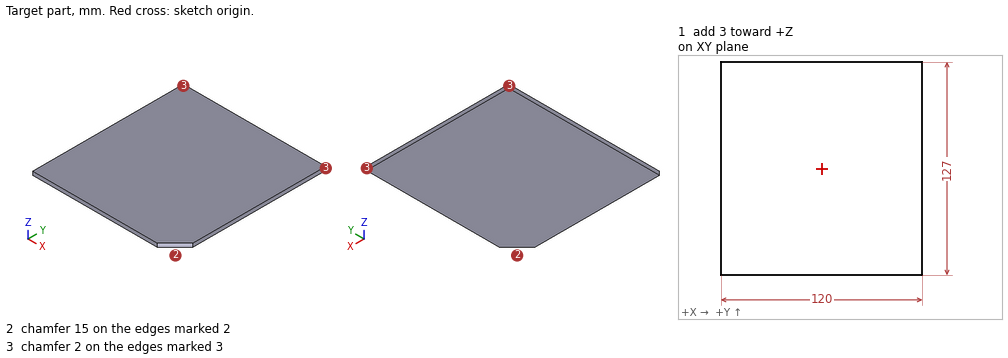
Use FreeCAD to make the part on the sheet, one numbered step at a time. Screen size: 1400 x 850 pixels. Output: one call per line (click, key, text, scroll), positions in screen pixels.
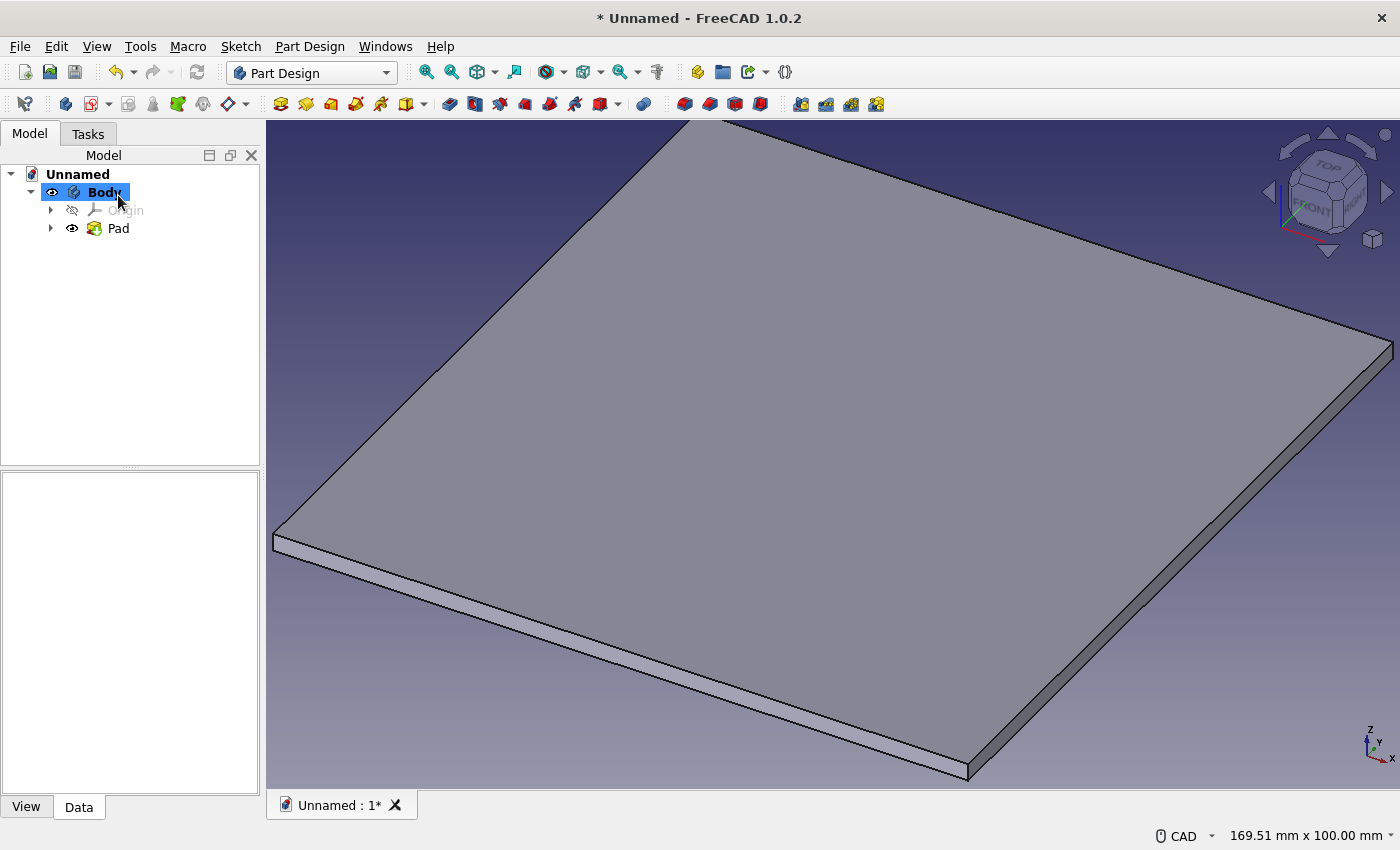
click(427, 72)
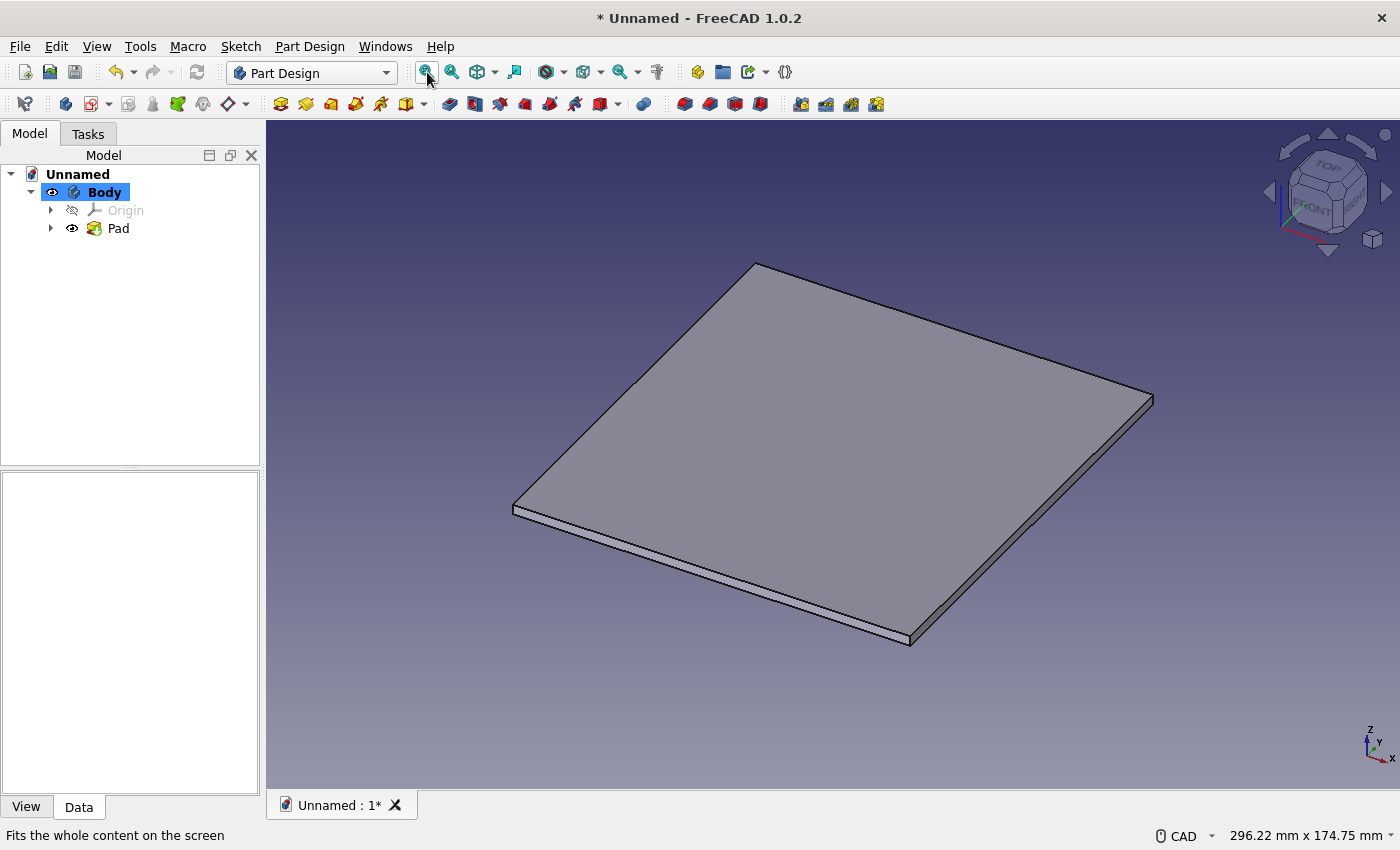
click(910, 642)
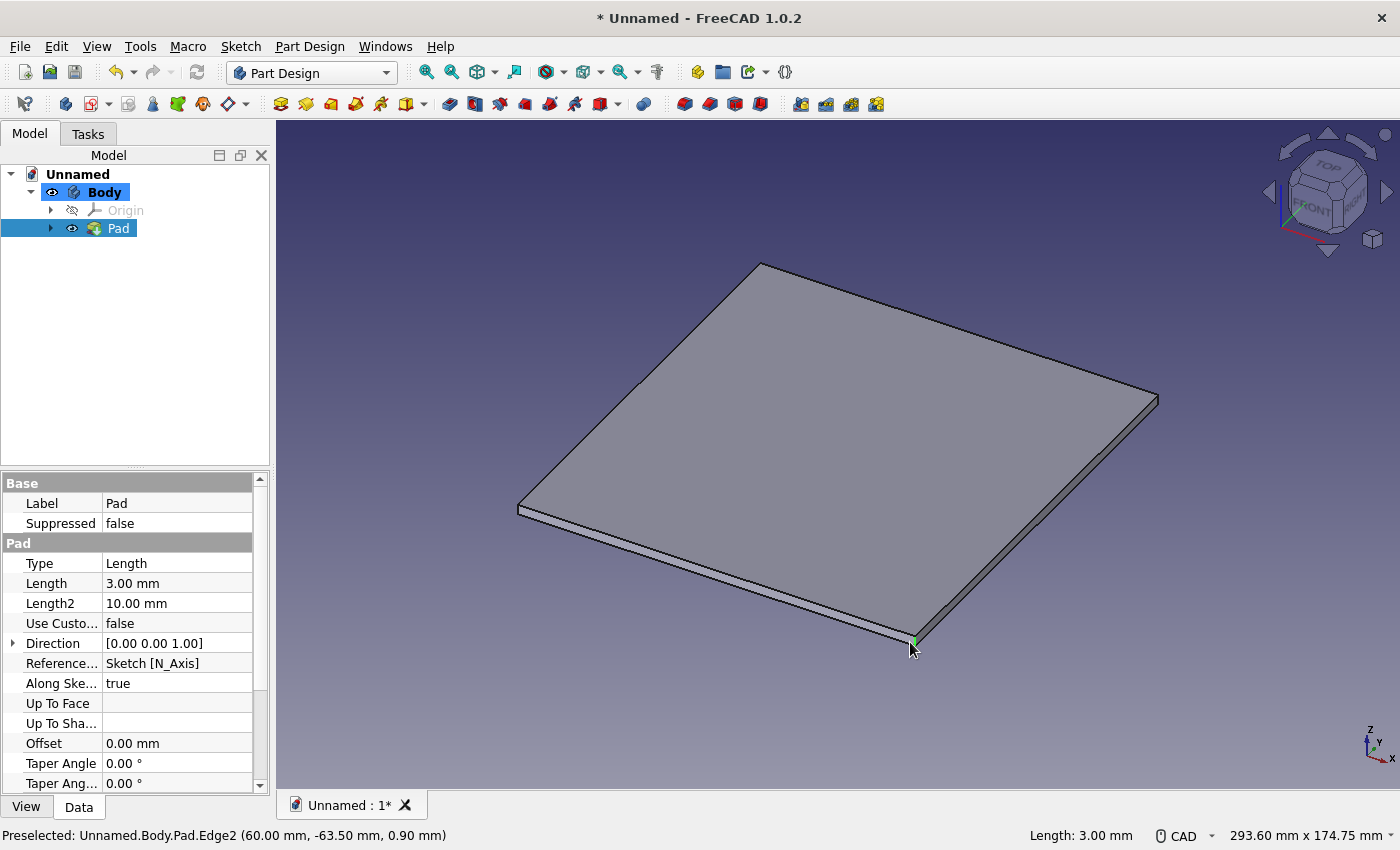
click(710, 104)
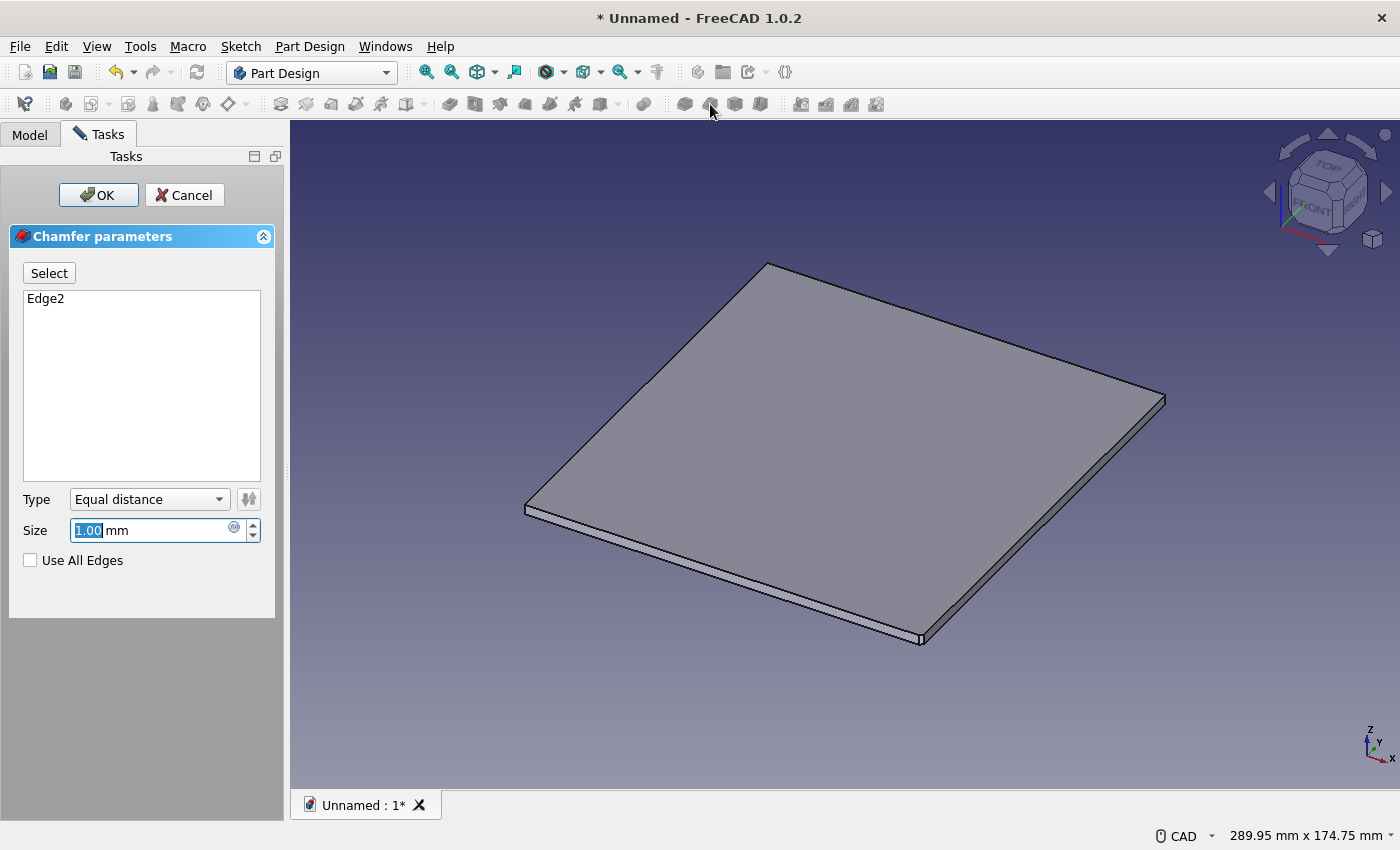
text(15)
key(Tab)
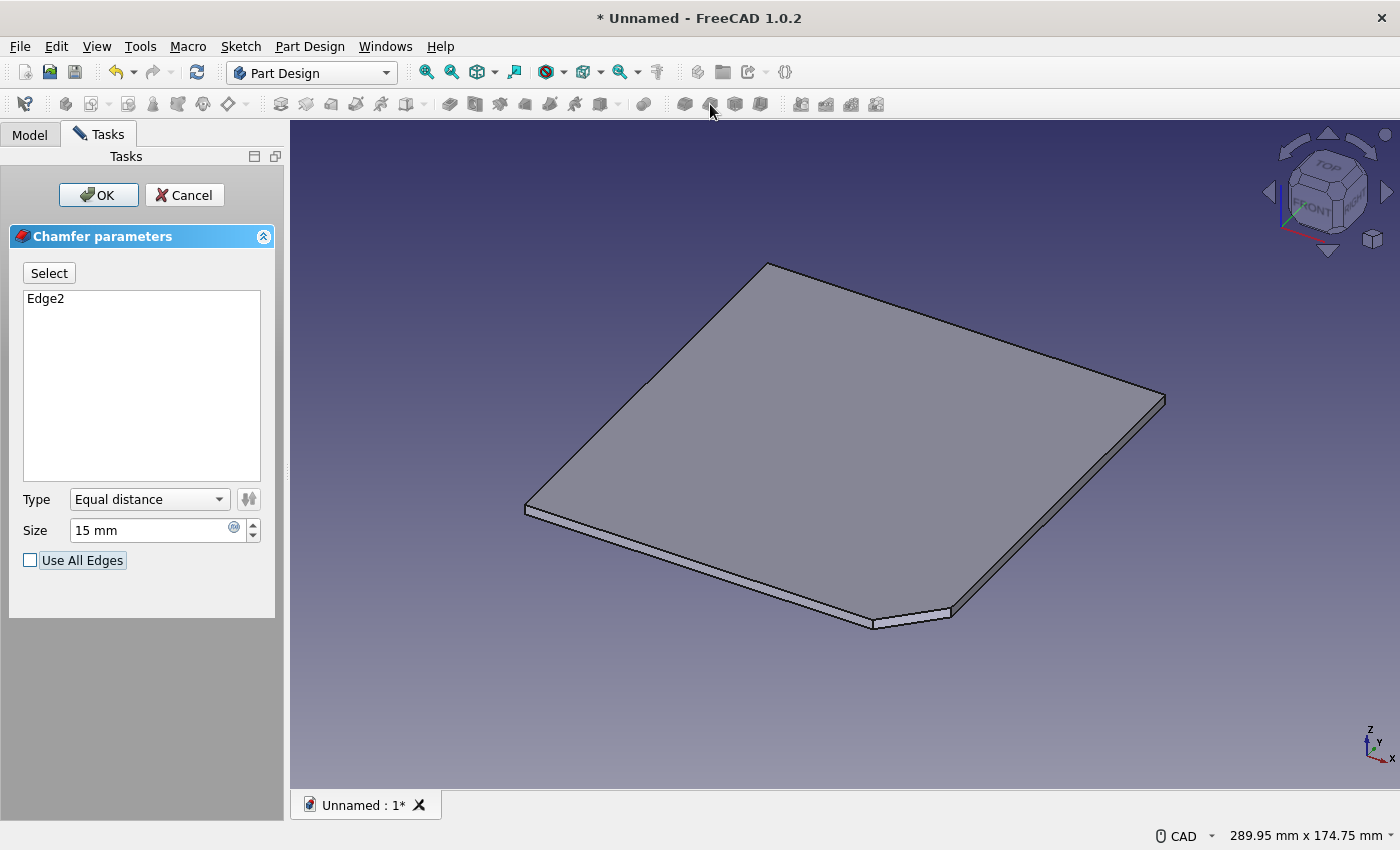
click(99, 195)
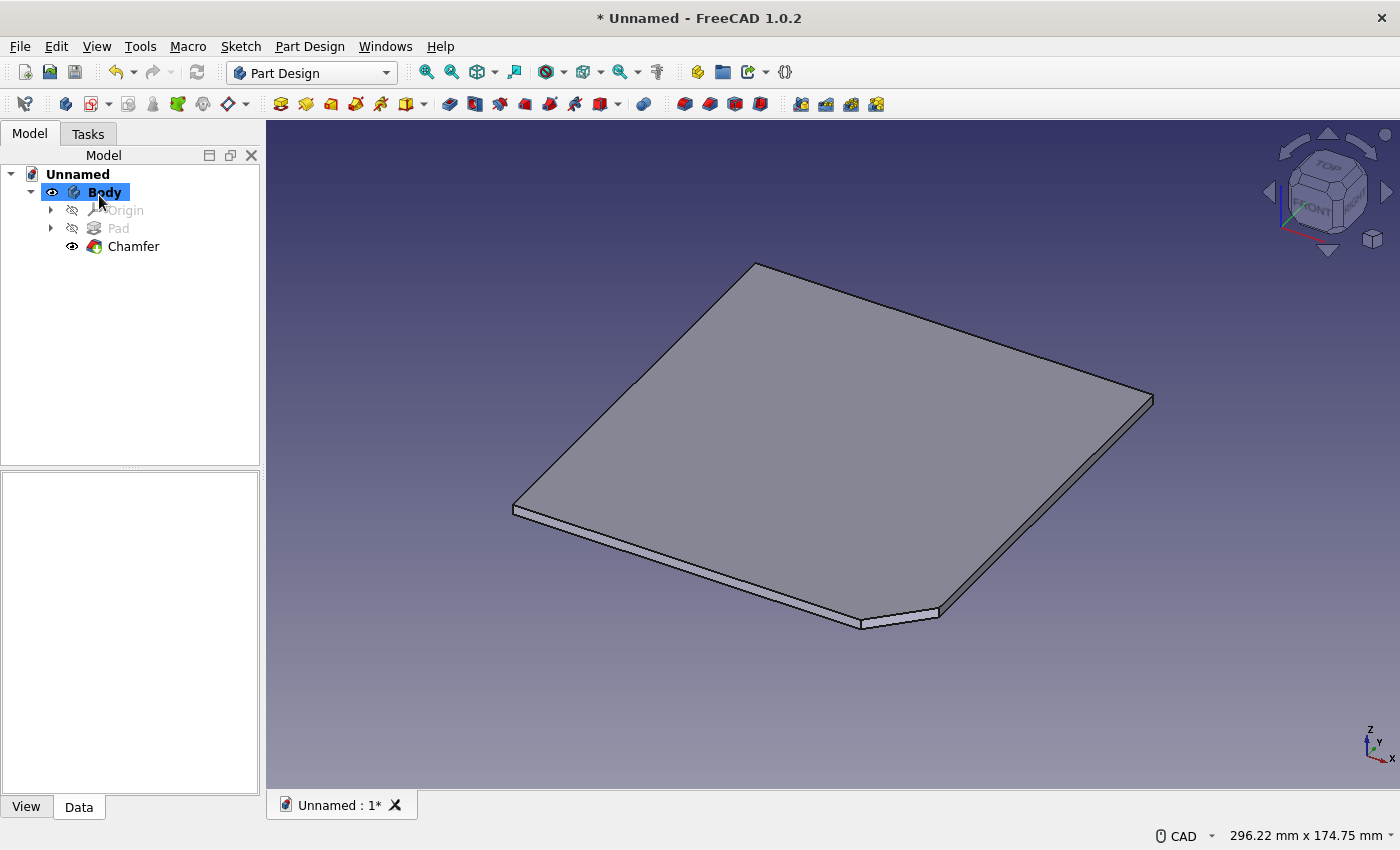
scroll(756, 267, up, 7)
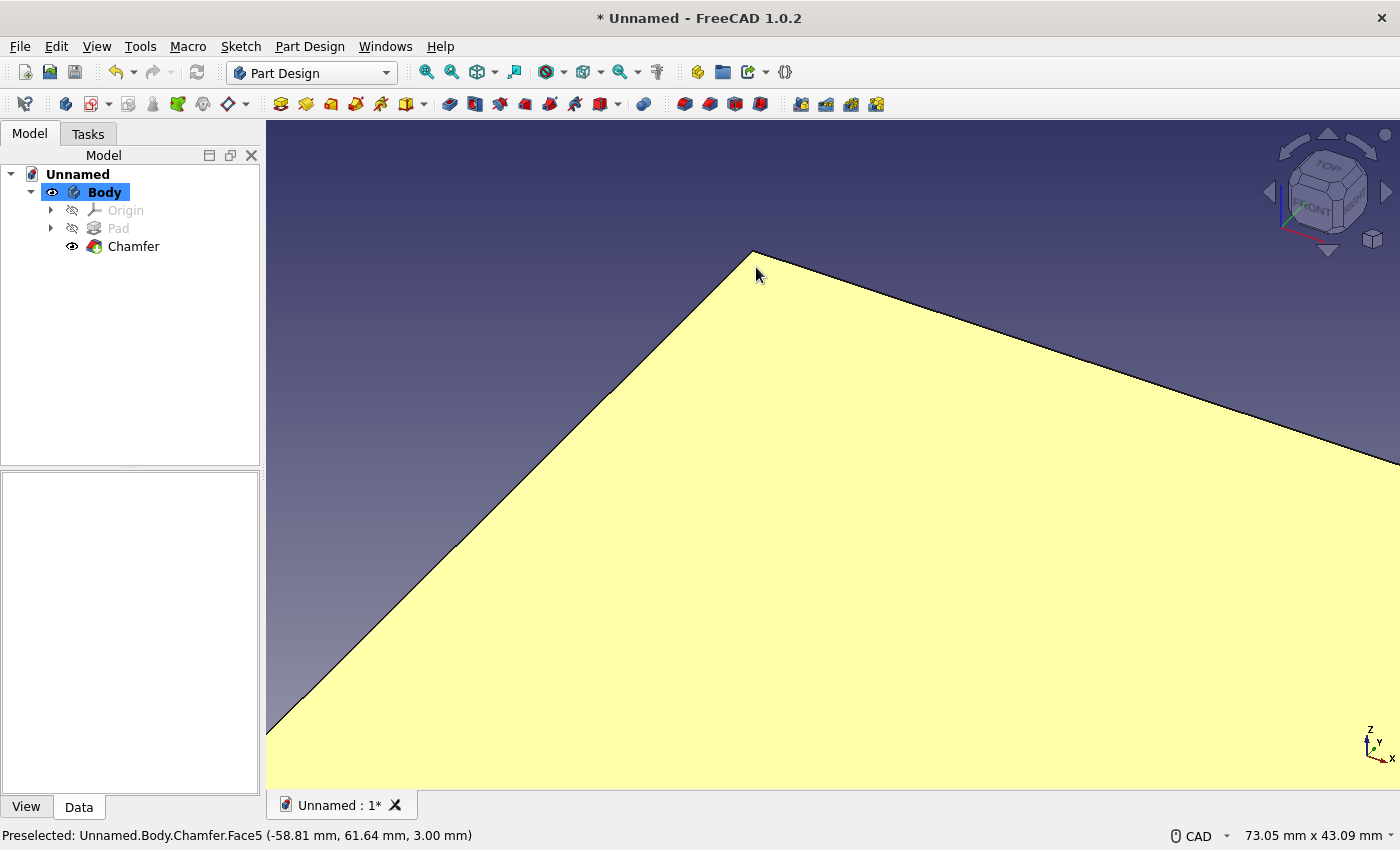
key(v)
key(f)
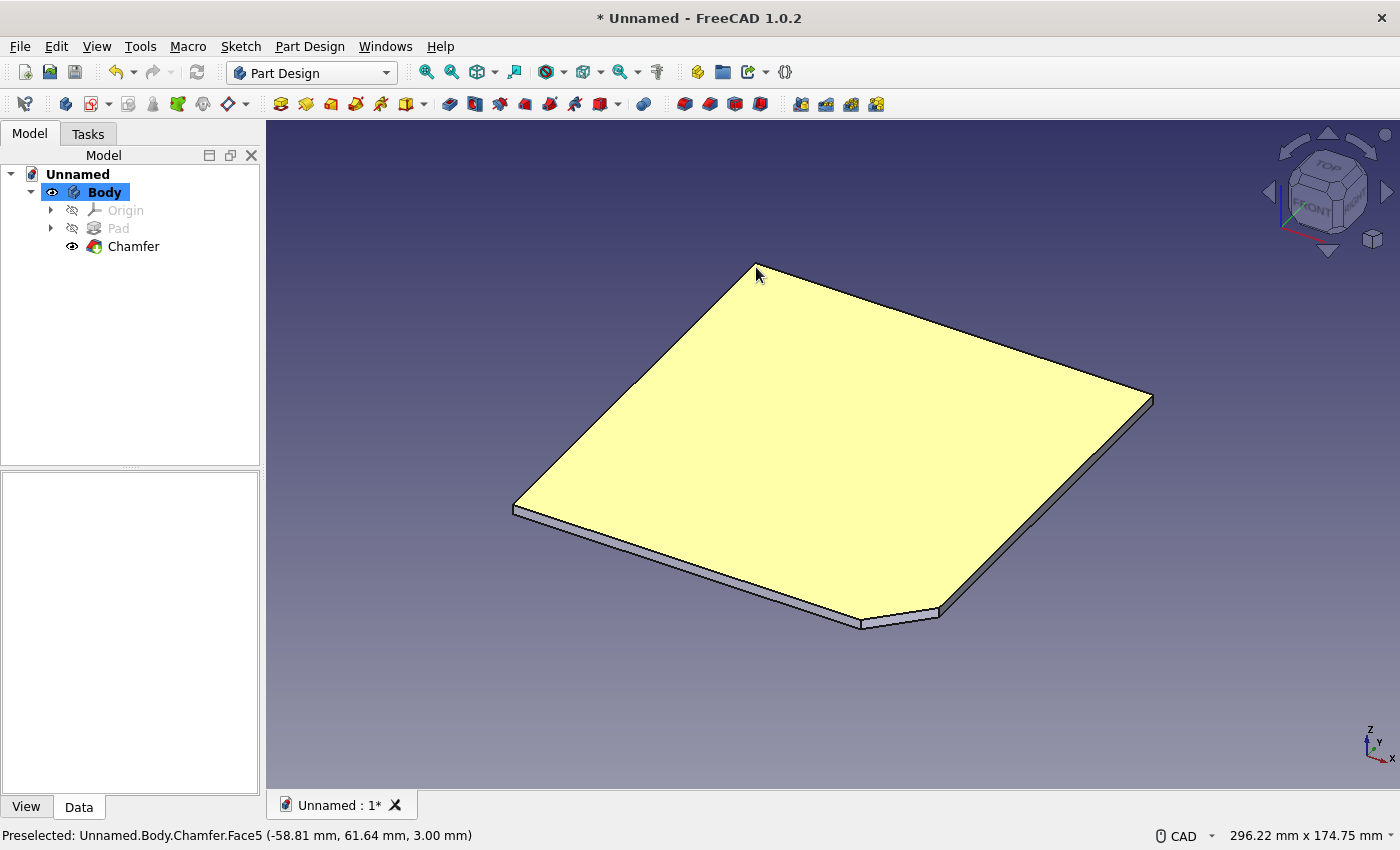
key(0)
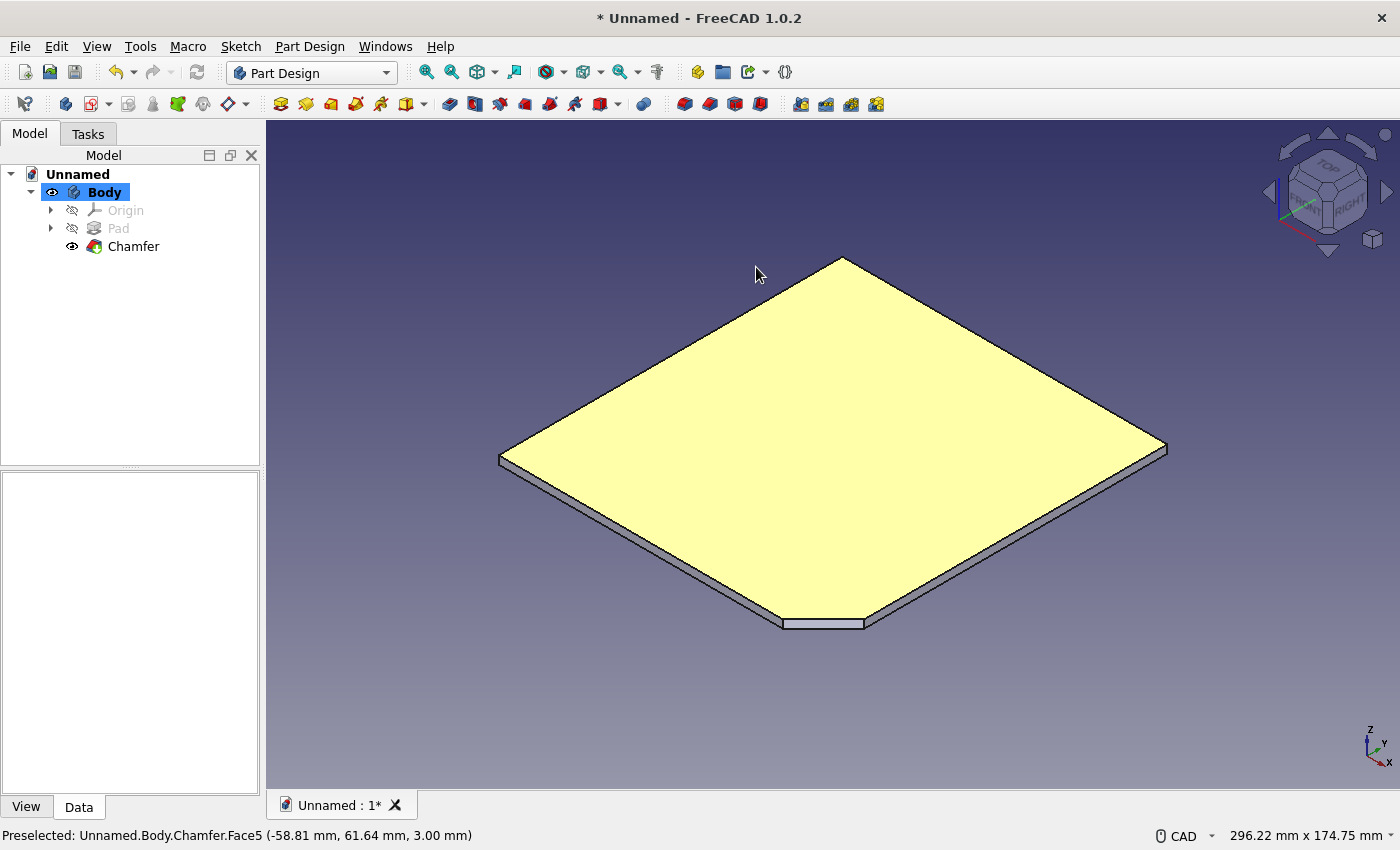
scroll(842, 260, up, 7)